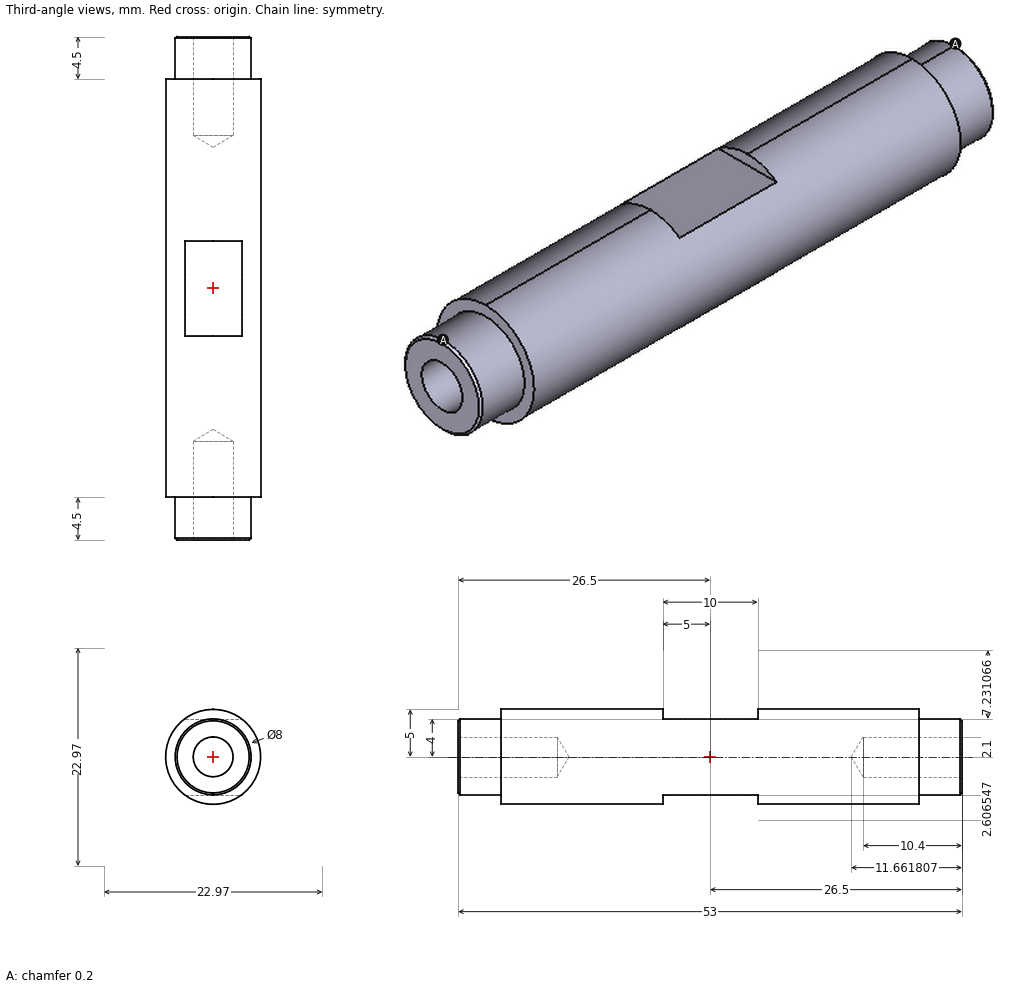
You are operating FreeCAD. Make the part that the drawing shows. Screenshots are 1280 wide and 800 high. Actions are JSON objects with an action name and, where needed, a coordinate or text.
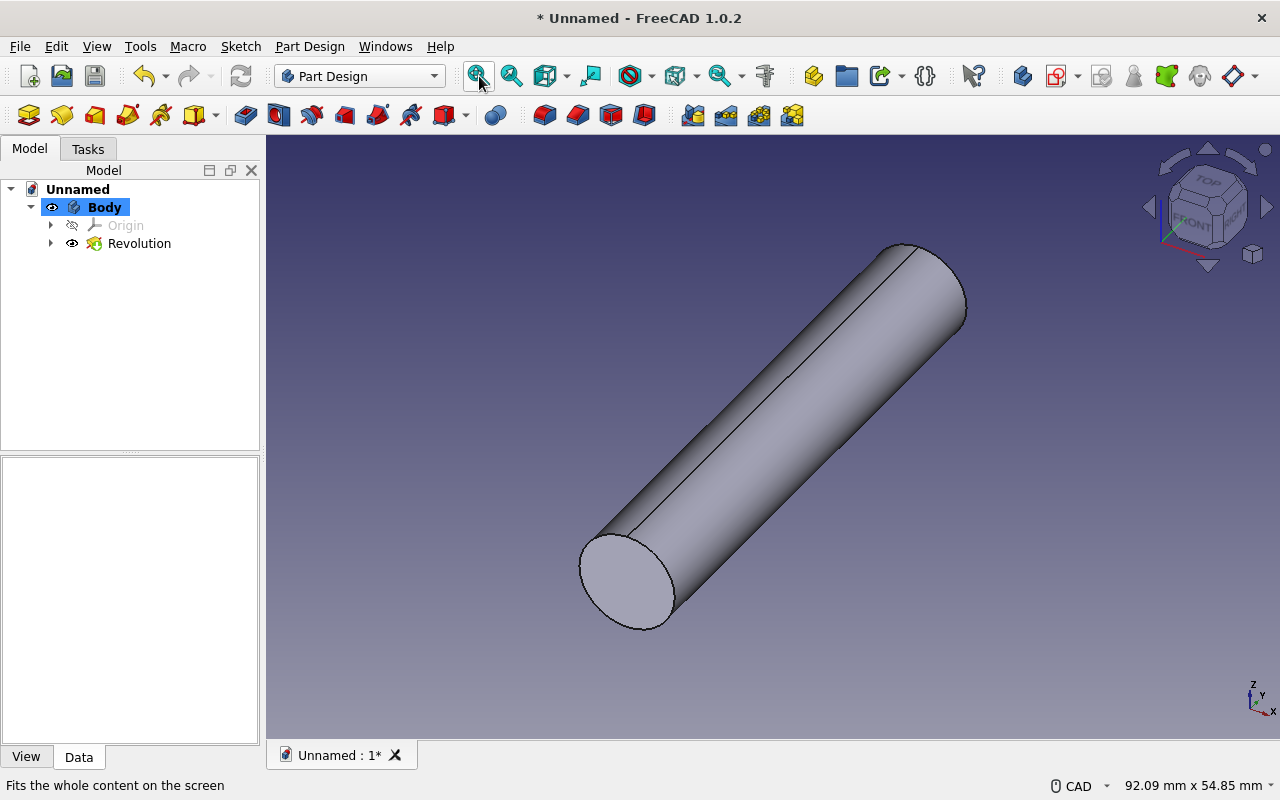
{"action": "left_click", "coordinate": [1056, 76]}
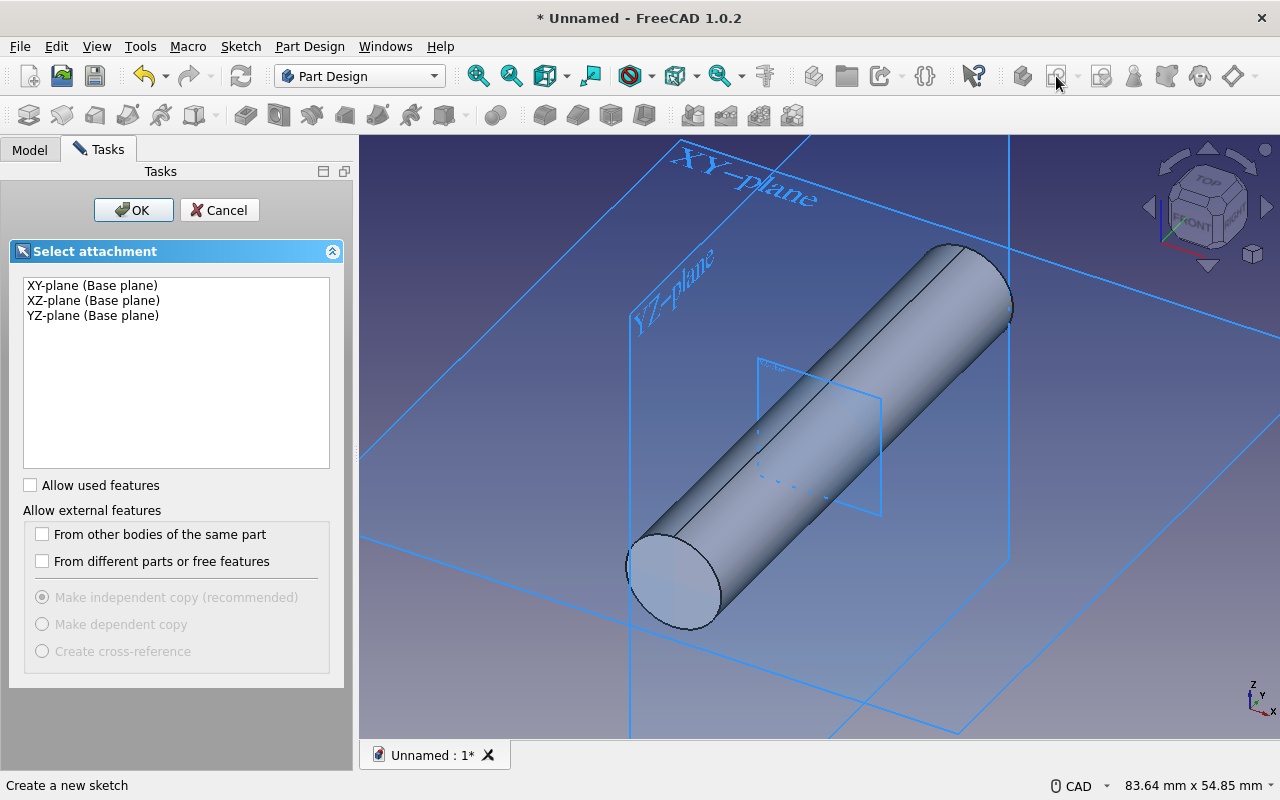
{"action": "left_click", "coordinate": [84, 316]}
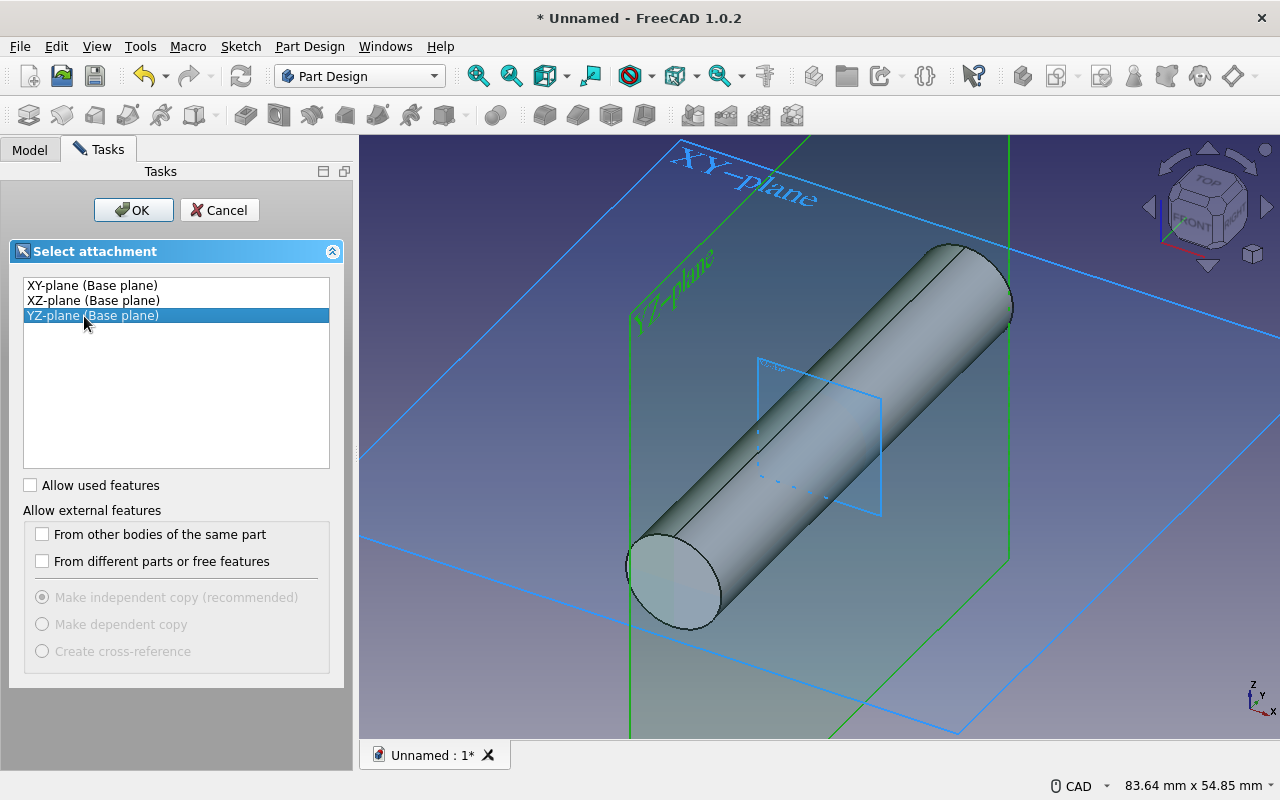
{"action": "left_click", "coordinate": [134, 210]}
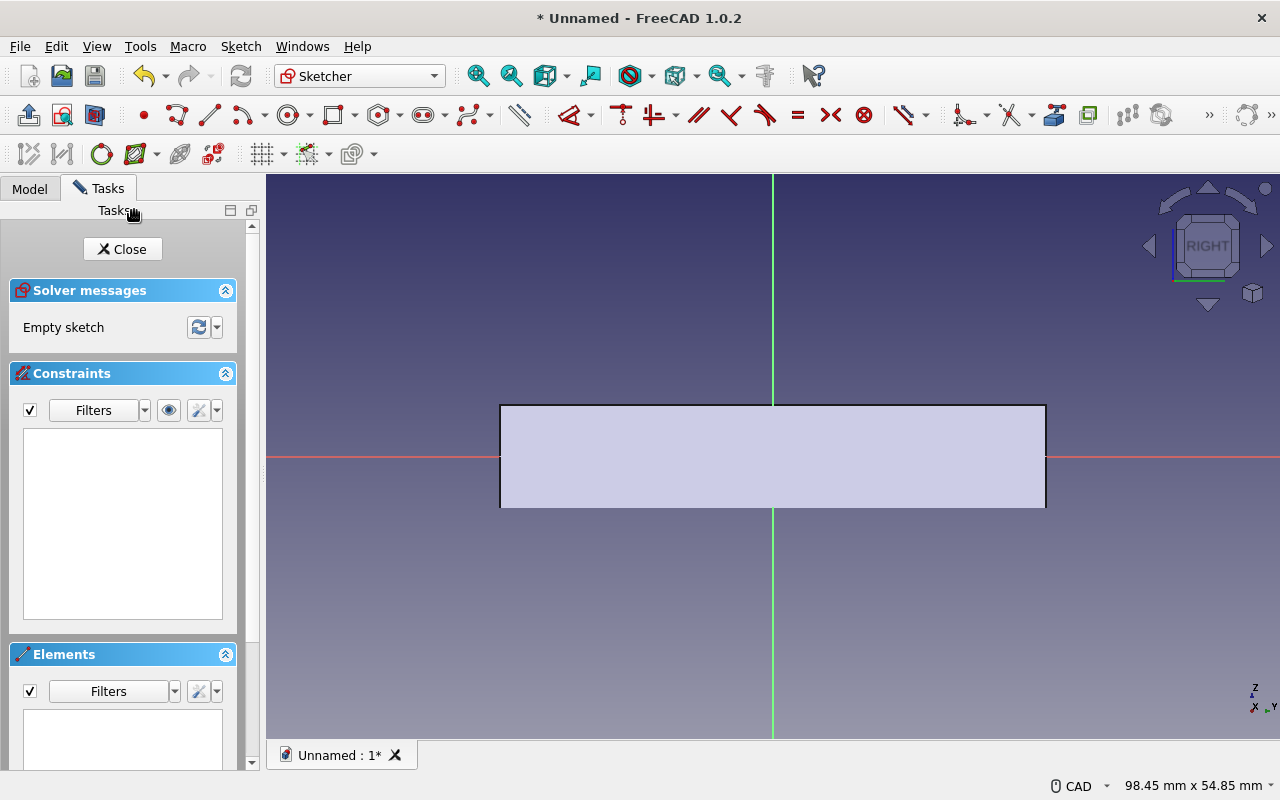
{"action": "left_click", "coordinate": [95, 116]}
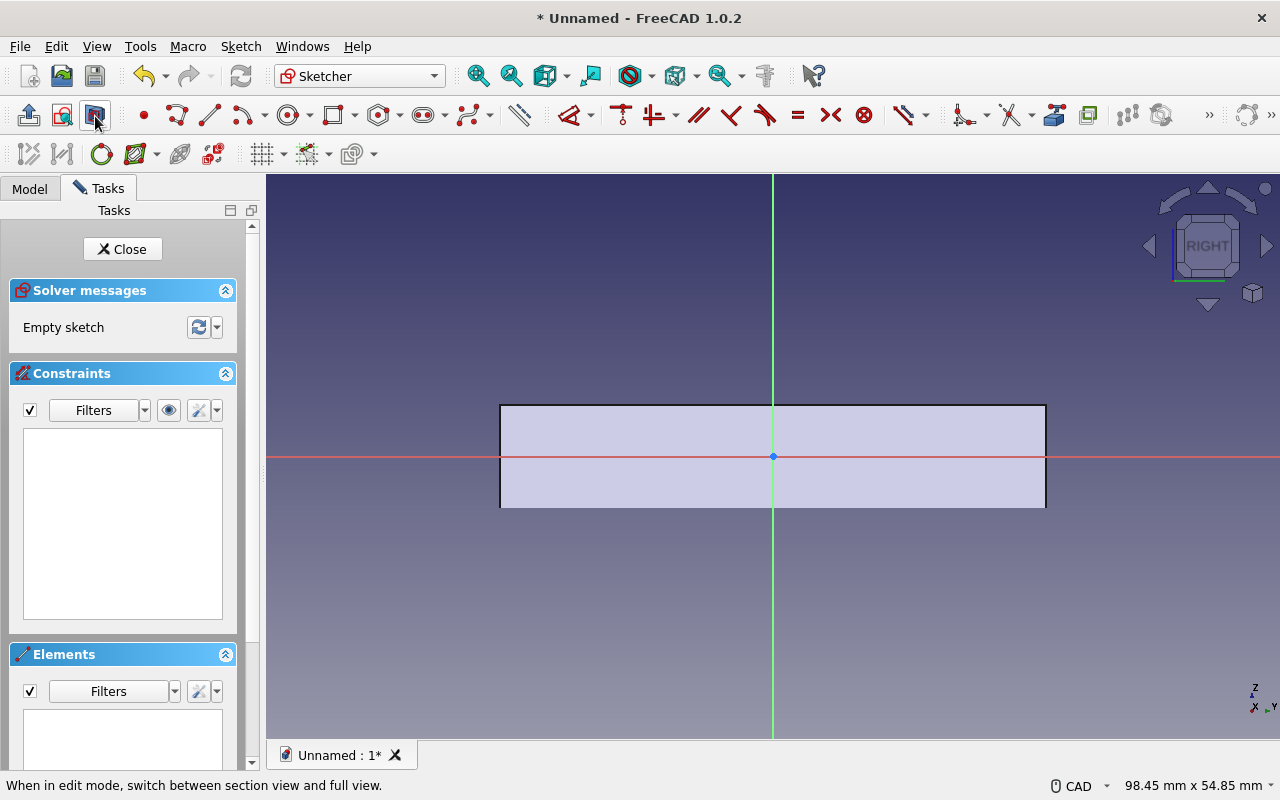
{"action": "scroll", "coordinate": [1077, 437], "scroll_direction": "up", "scroll_amount": 4}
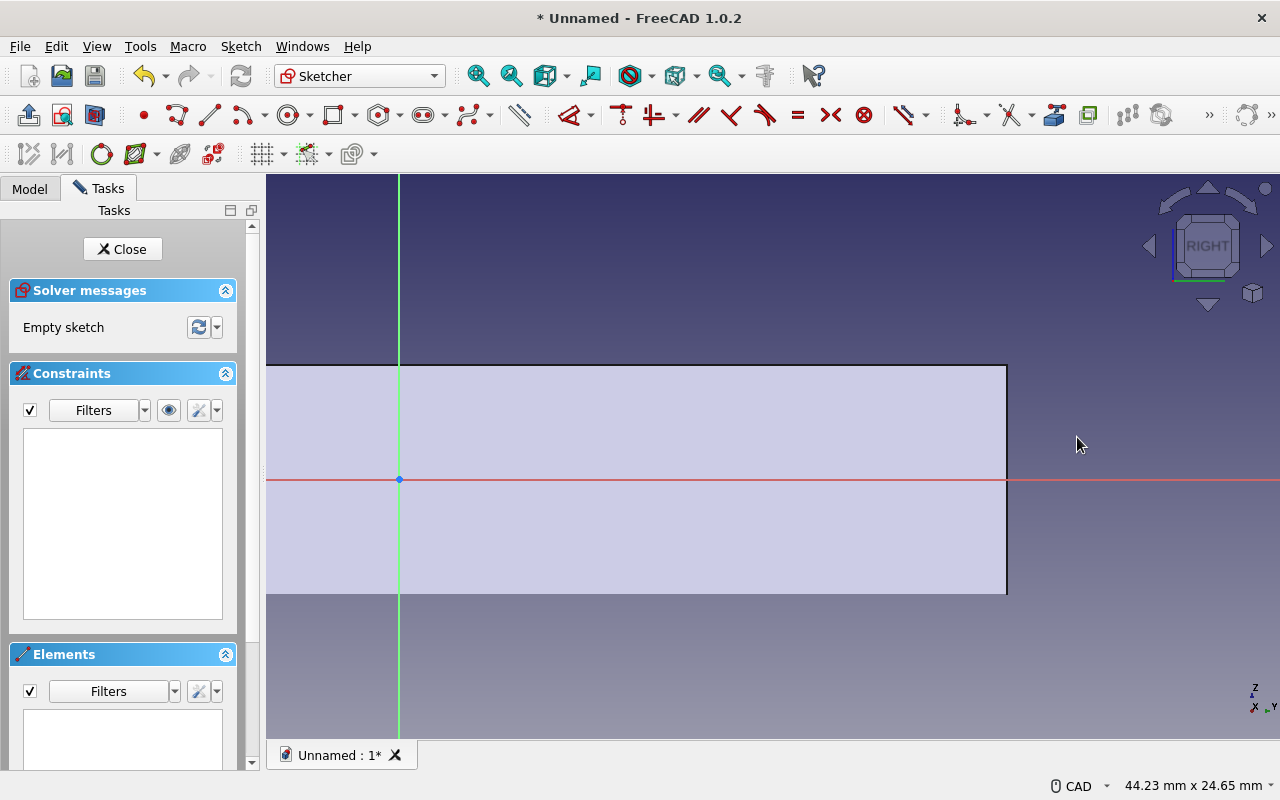
{"action": "left_click", "coordinate": [177, 116]}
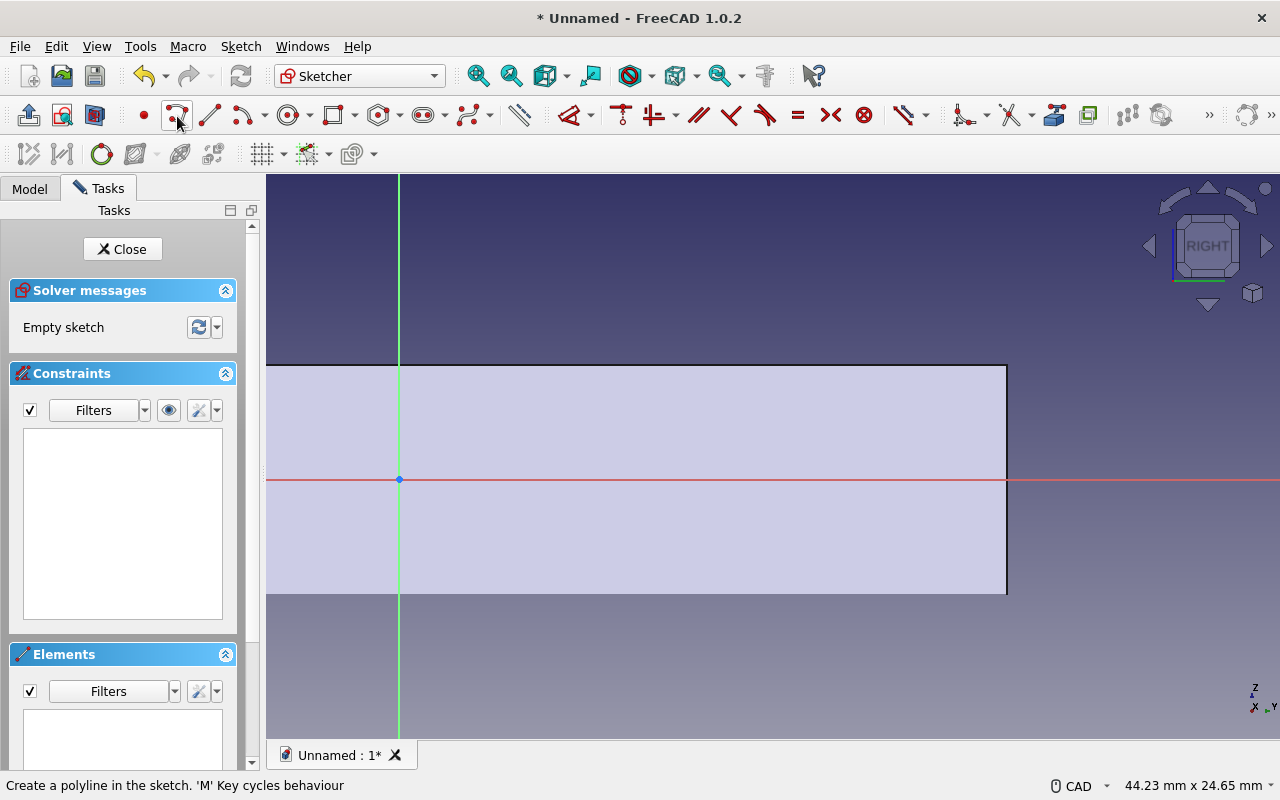
{"action": "left_click", "coordinate": [740, 480]}
{"action": "left_click", "coordinate": [1007, 471]}
{"action": "left_click", "coordinate": [1007, 432]}
{"action": "left_click", "coordinate": [769, 432]}
{"action": "left_click", "coordinate": [740, 480]}
{"action": "key", "text": "Escape"}
{"action": "key", "text": "Escape"}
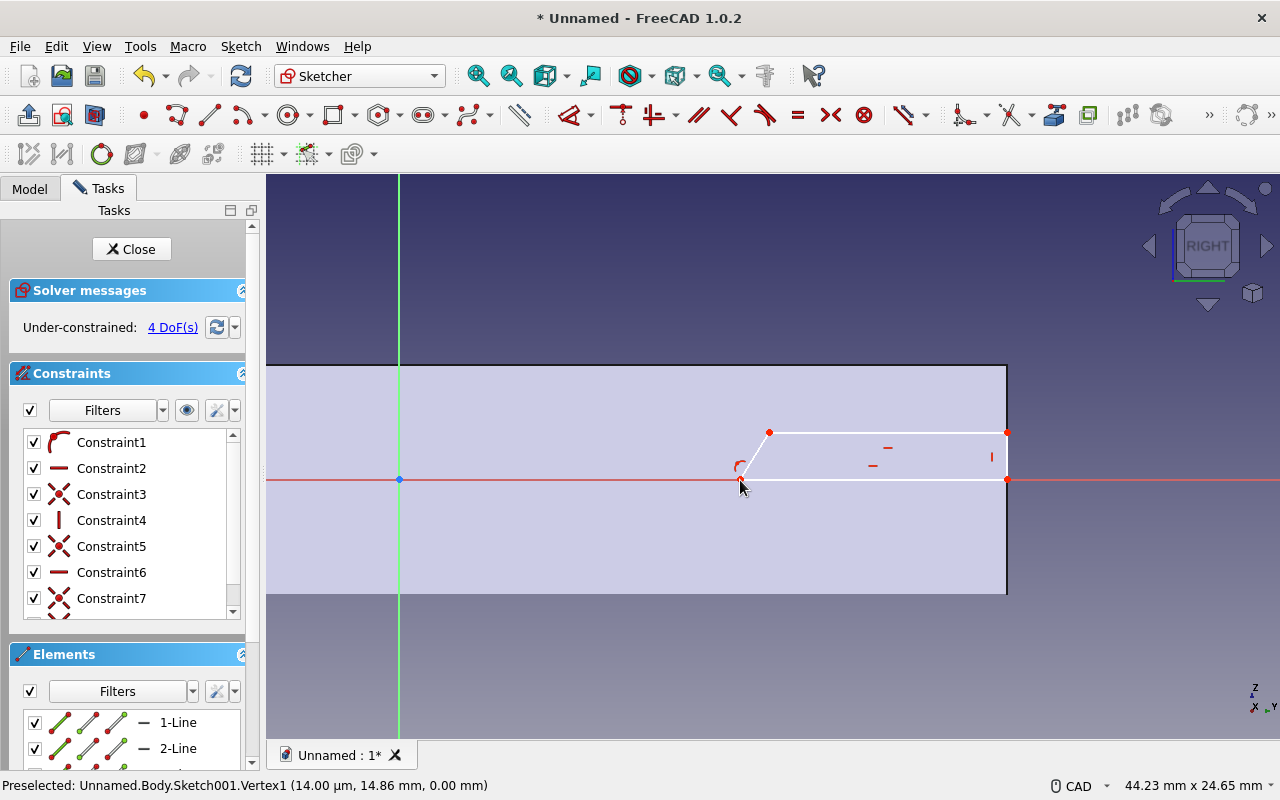
{"action": "left_click", "coordinate": [568, 116]}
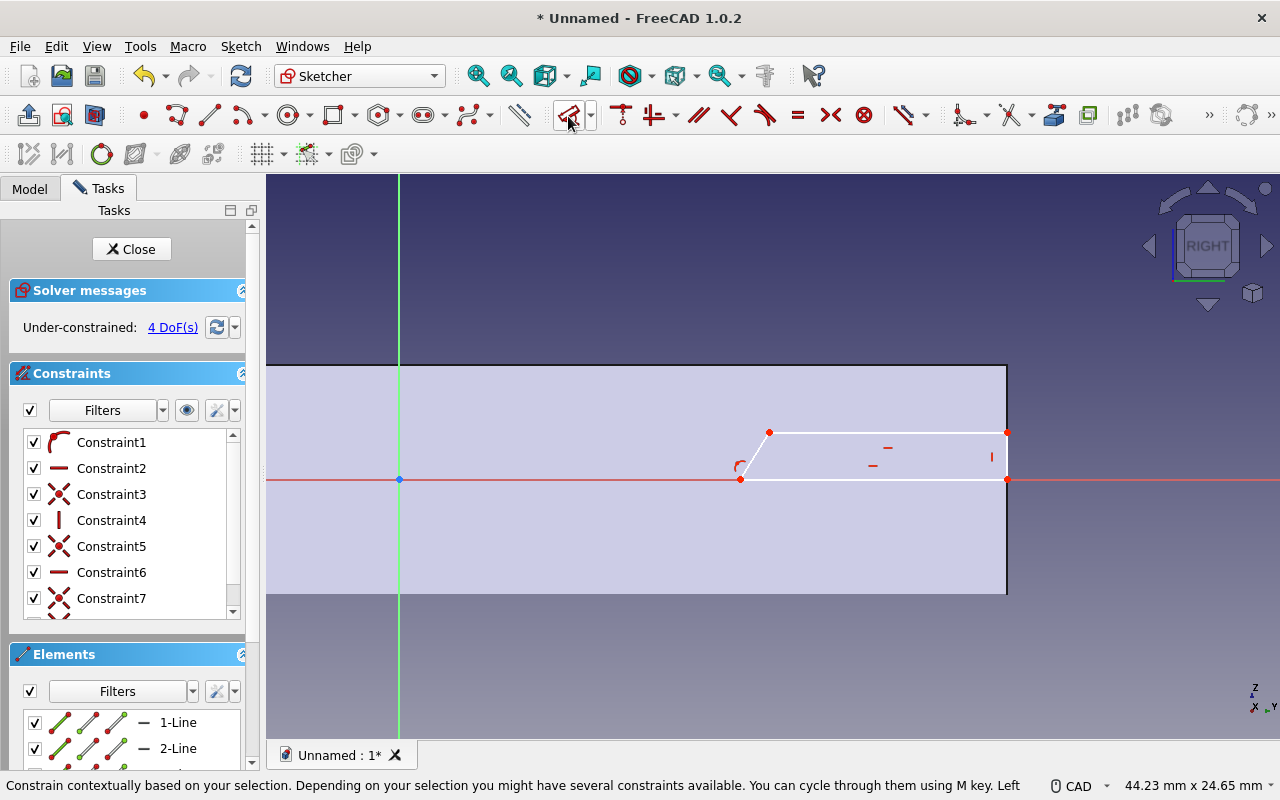
{"action": "left_click", "coordinate": [1007, 466]}
{"action": "left_click", "coordinate": [1041, 456]}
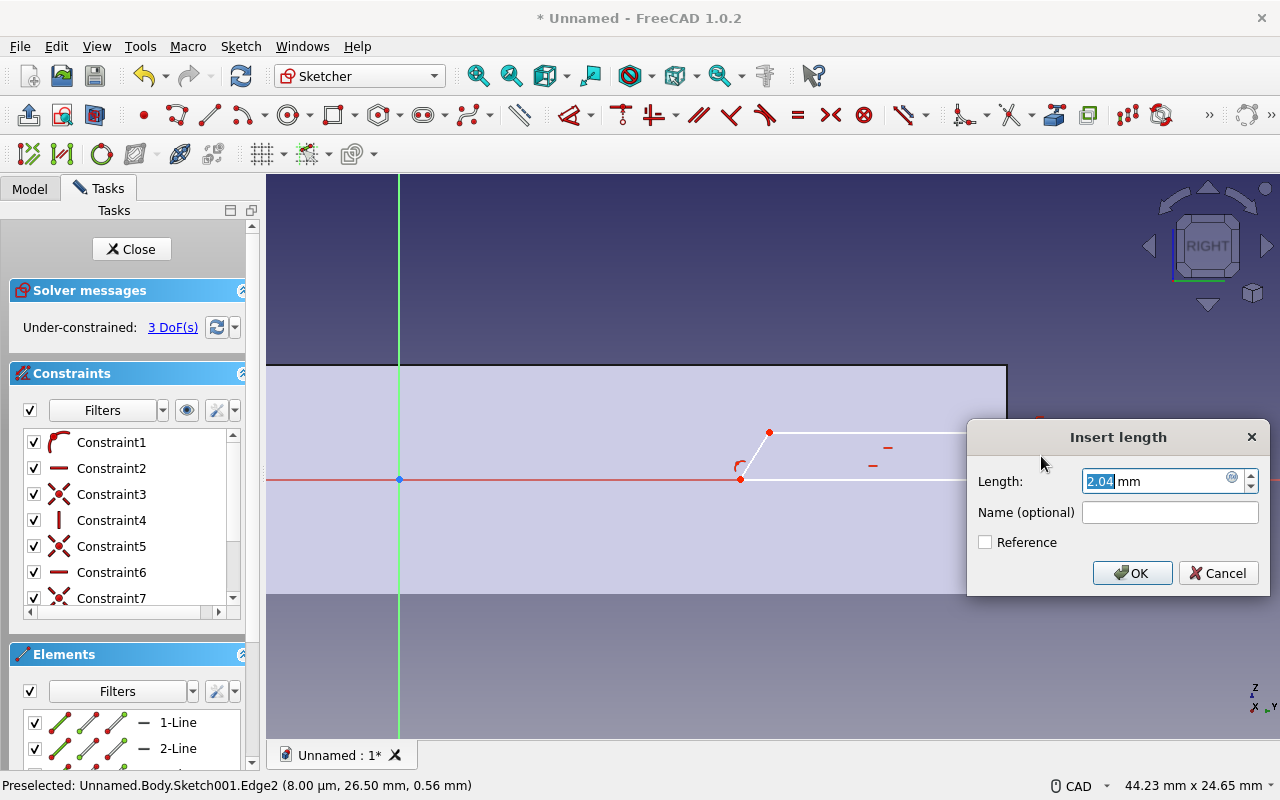
{"action": "type", "text": "2.1"}
{"action": "key", "text": "Return"}